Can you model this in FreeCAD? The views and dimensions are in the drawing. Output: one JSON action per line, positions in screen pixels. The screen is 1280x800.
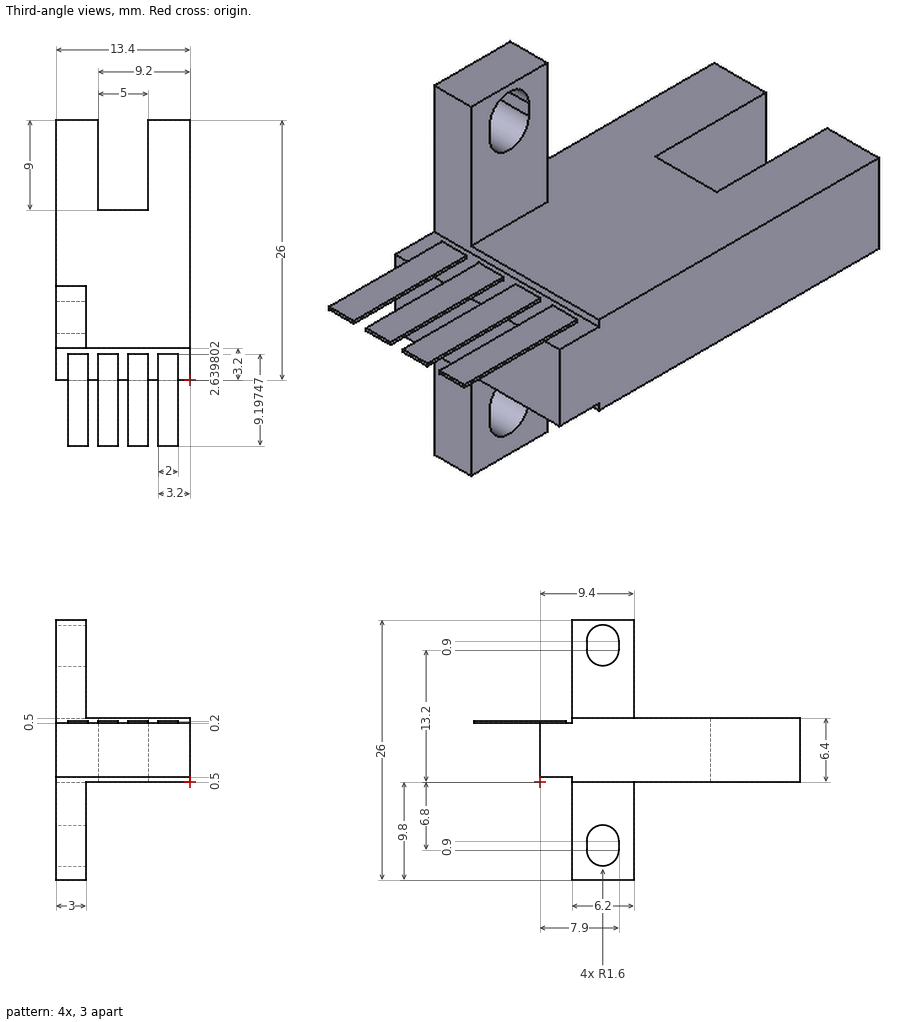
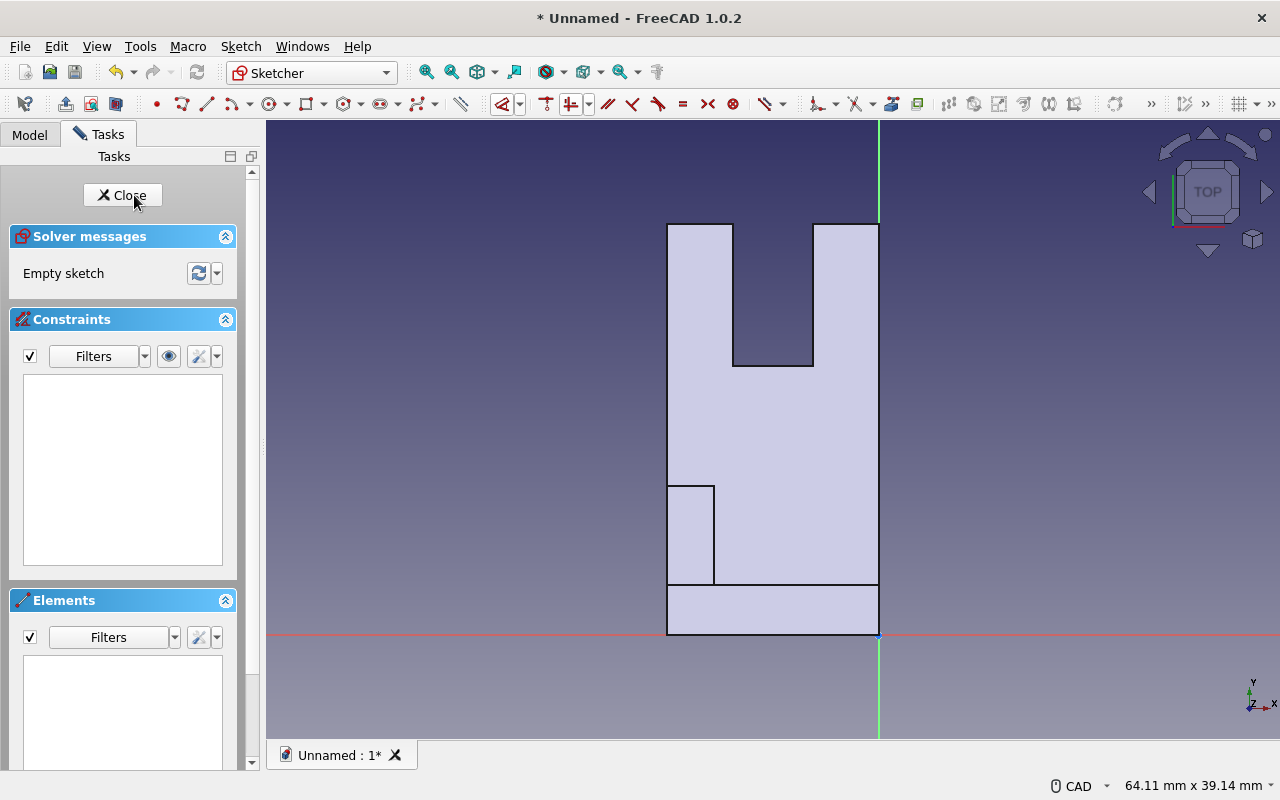
{"action": "left_click", "coordinate": [116, 104]}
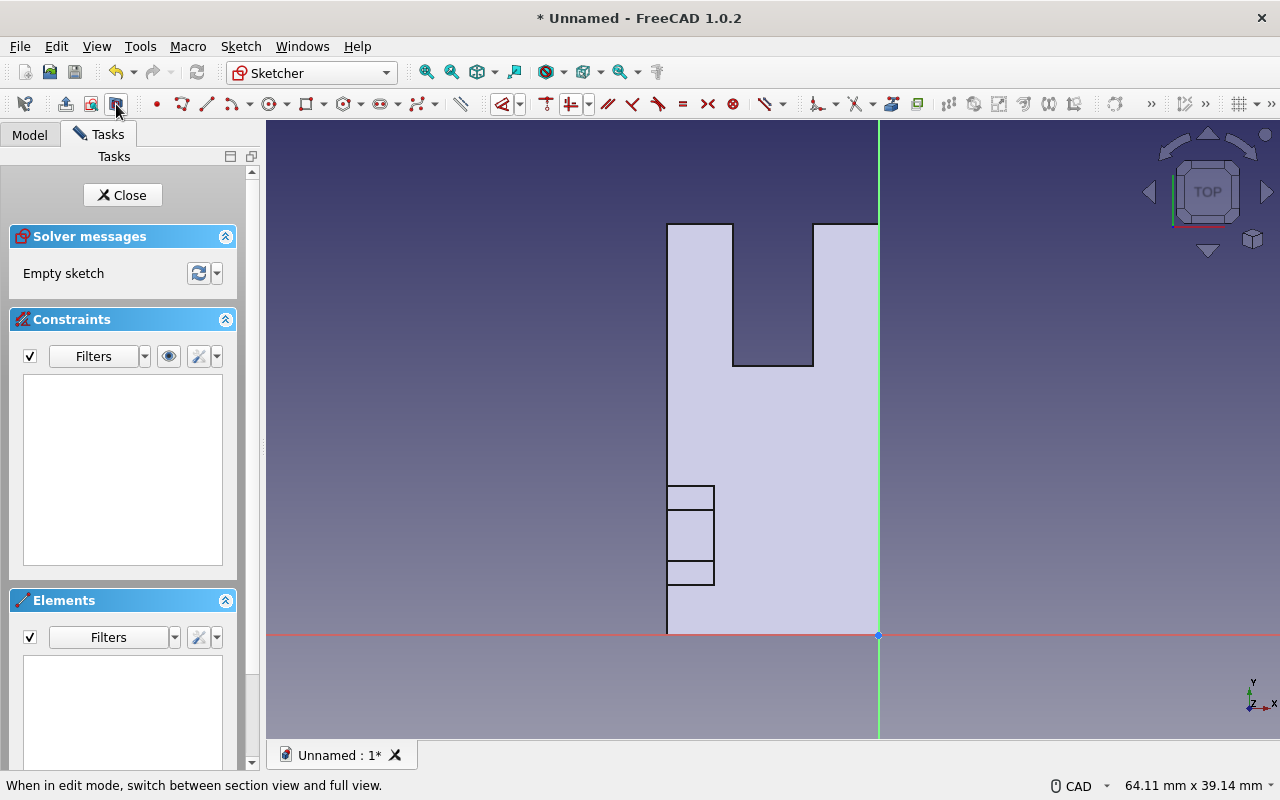
{"action": "scroll", "coordinate": [813, 711], "scroll_direction": "up", "scroll_amount": 5}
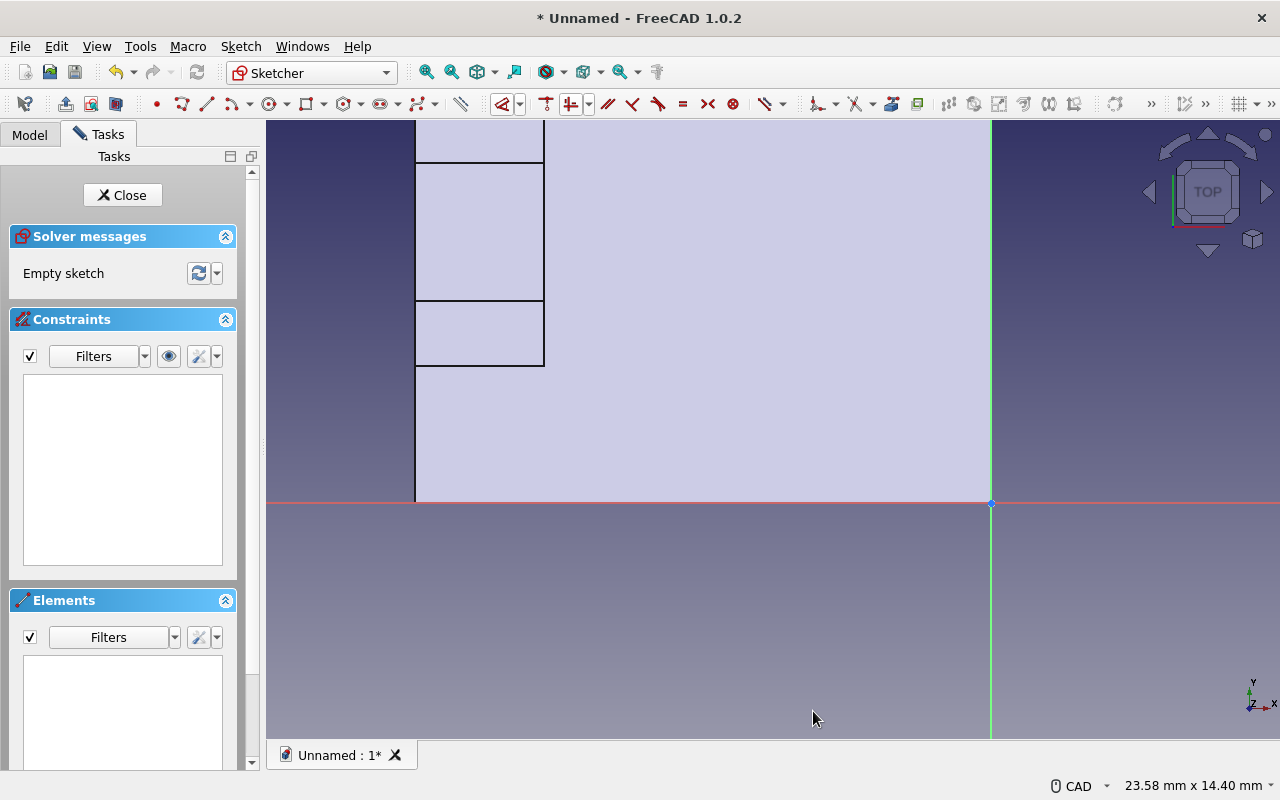
{"action": "left_click", "coordinate": [306, 104]}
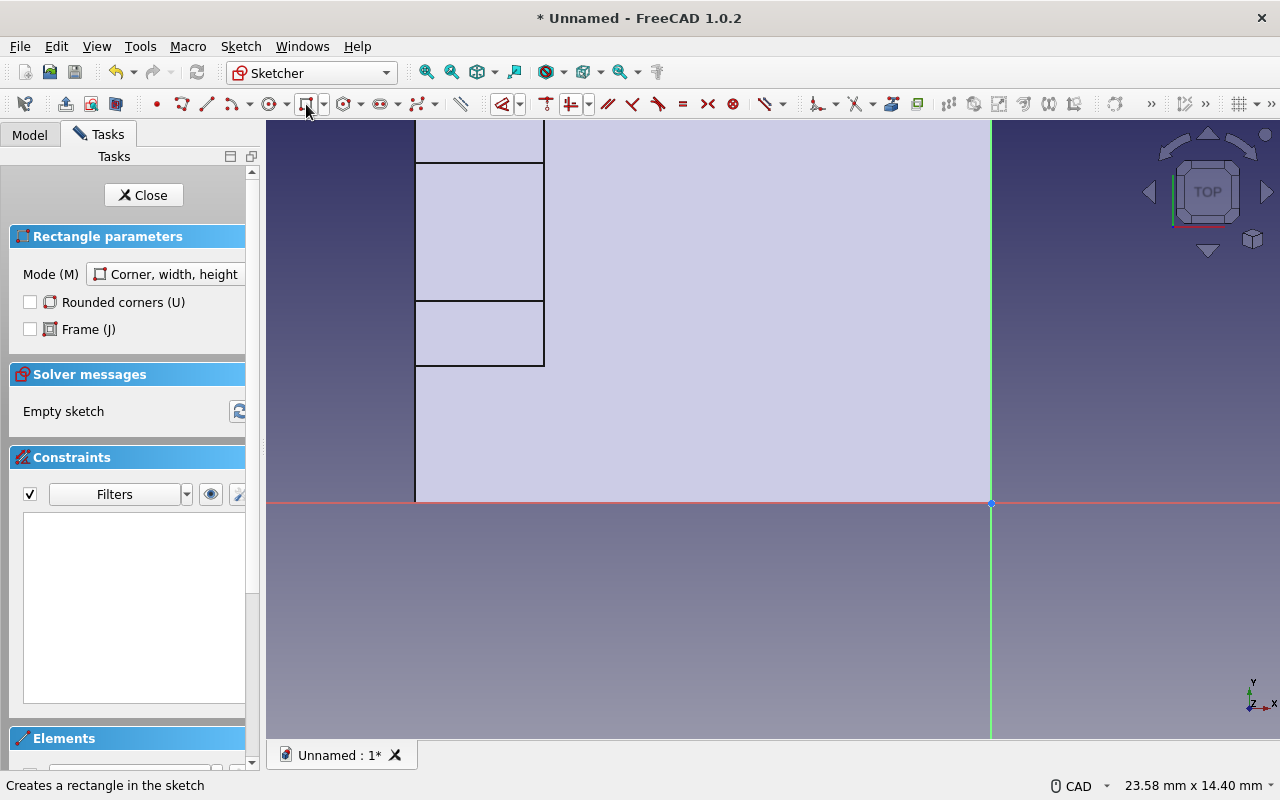
{"action": "left_click", "coordinate": [991, 503]}
{"action": "left_click", "coordinate": [415, 366]}
{"action": "key", "text": "Escape"}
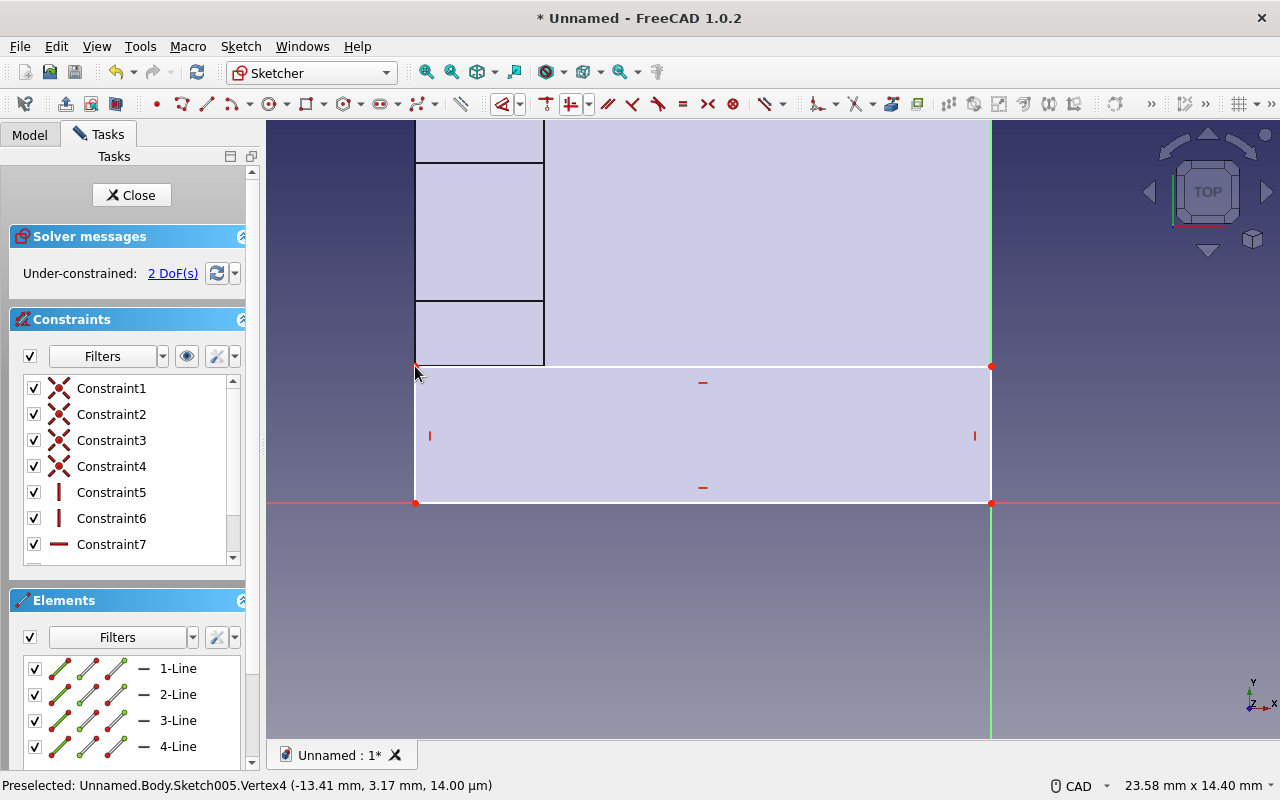
{"action": "left_click", "coordinate": [991, 462]}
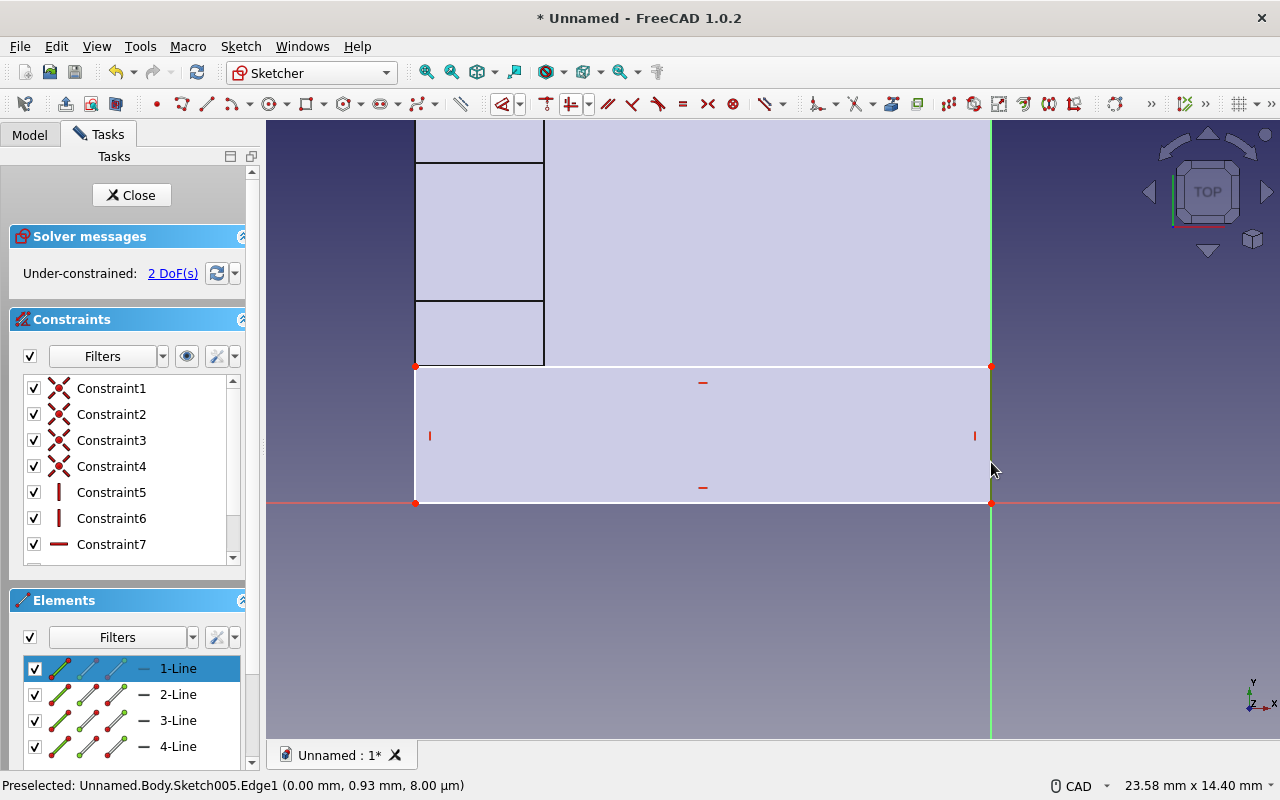
{"action": "left_click", "coordinate": [520, 104]}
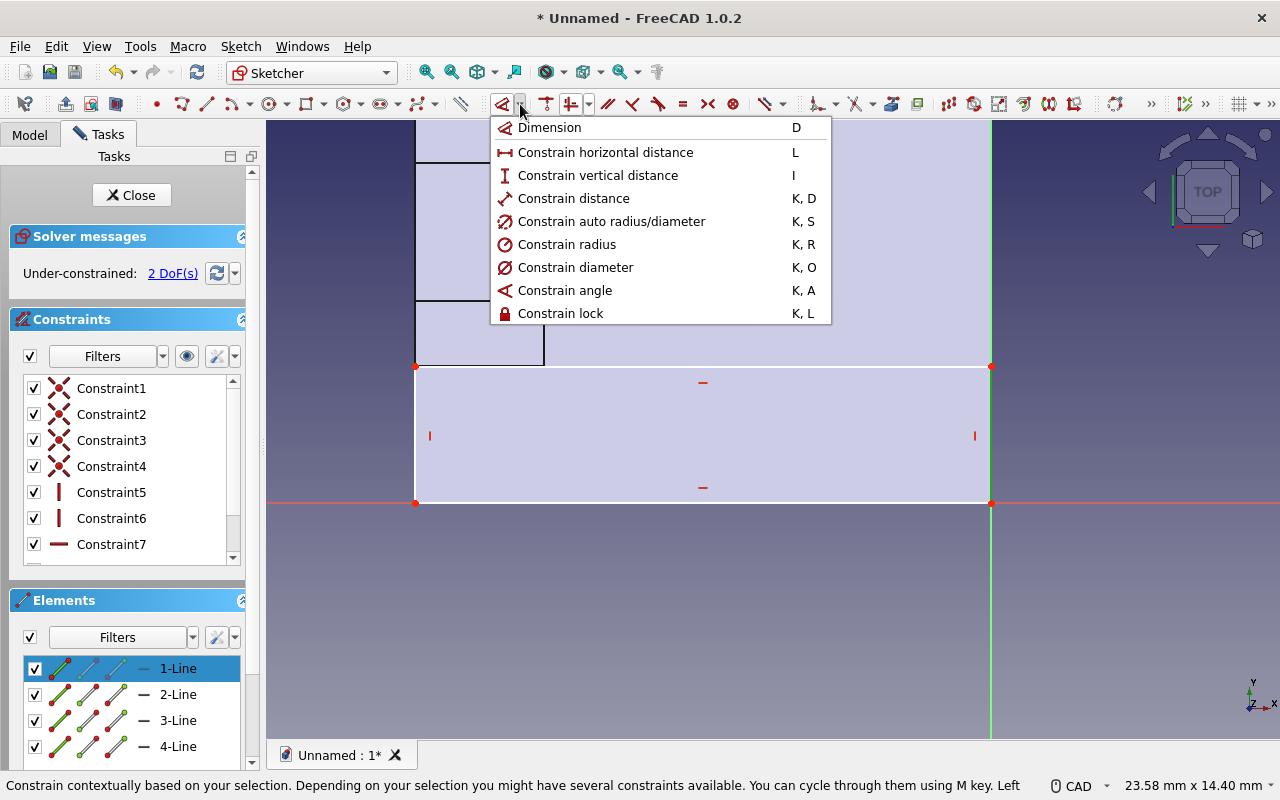
{"action": "left_click", "coordinate": [661, 176]}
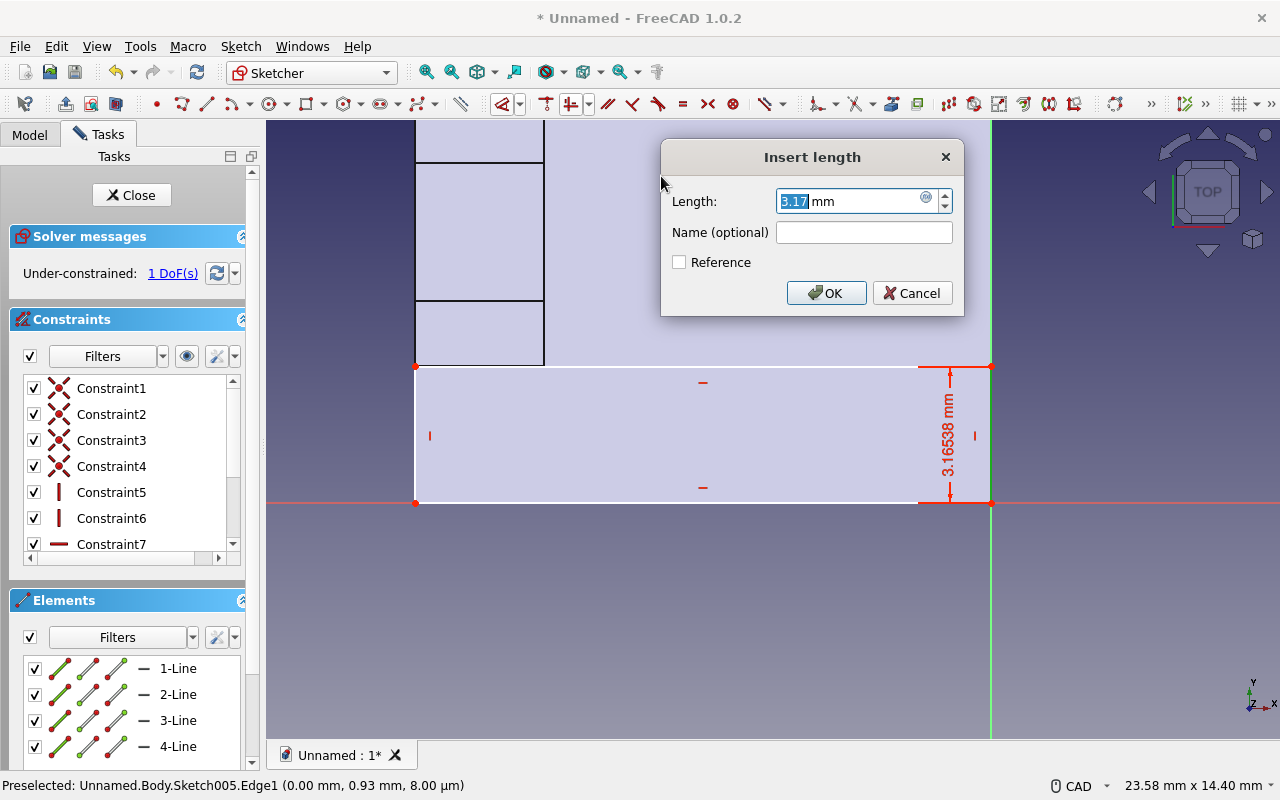
{"action": "type", "text": "3.2"}
{"action": "key", "text": "Return"}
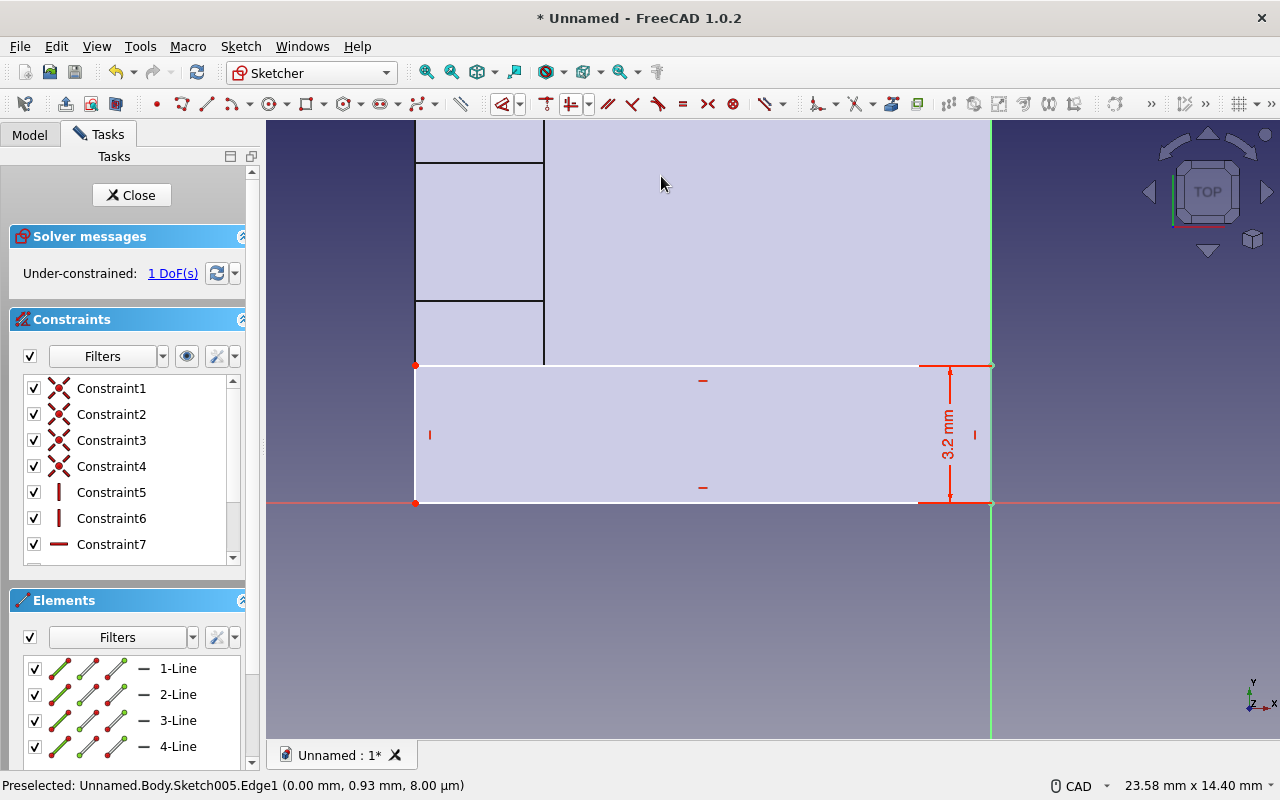
{"action": "left_click", "coordinate": [818, 366]}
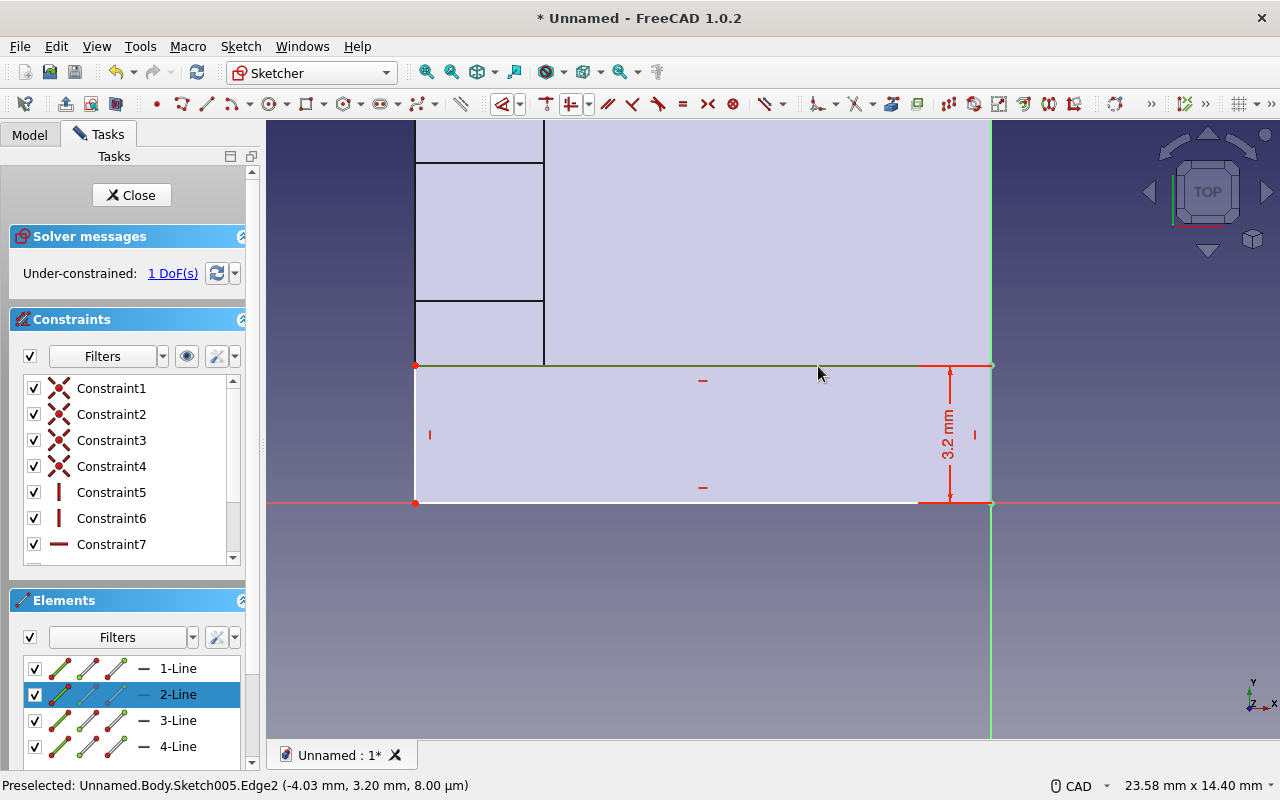
{"action": "left_click", "coordinate": [520, 104]}